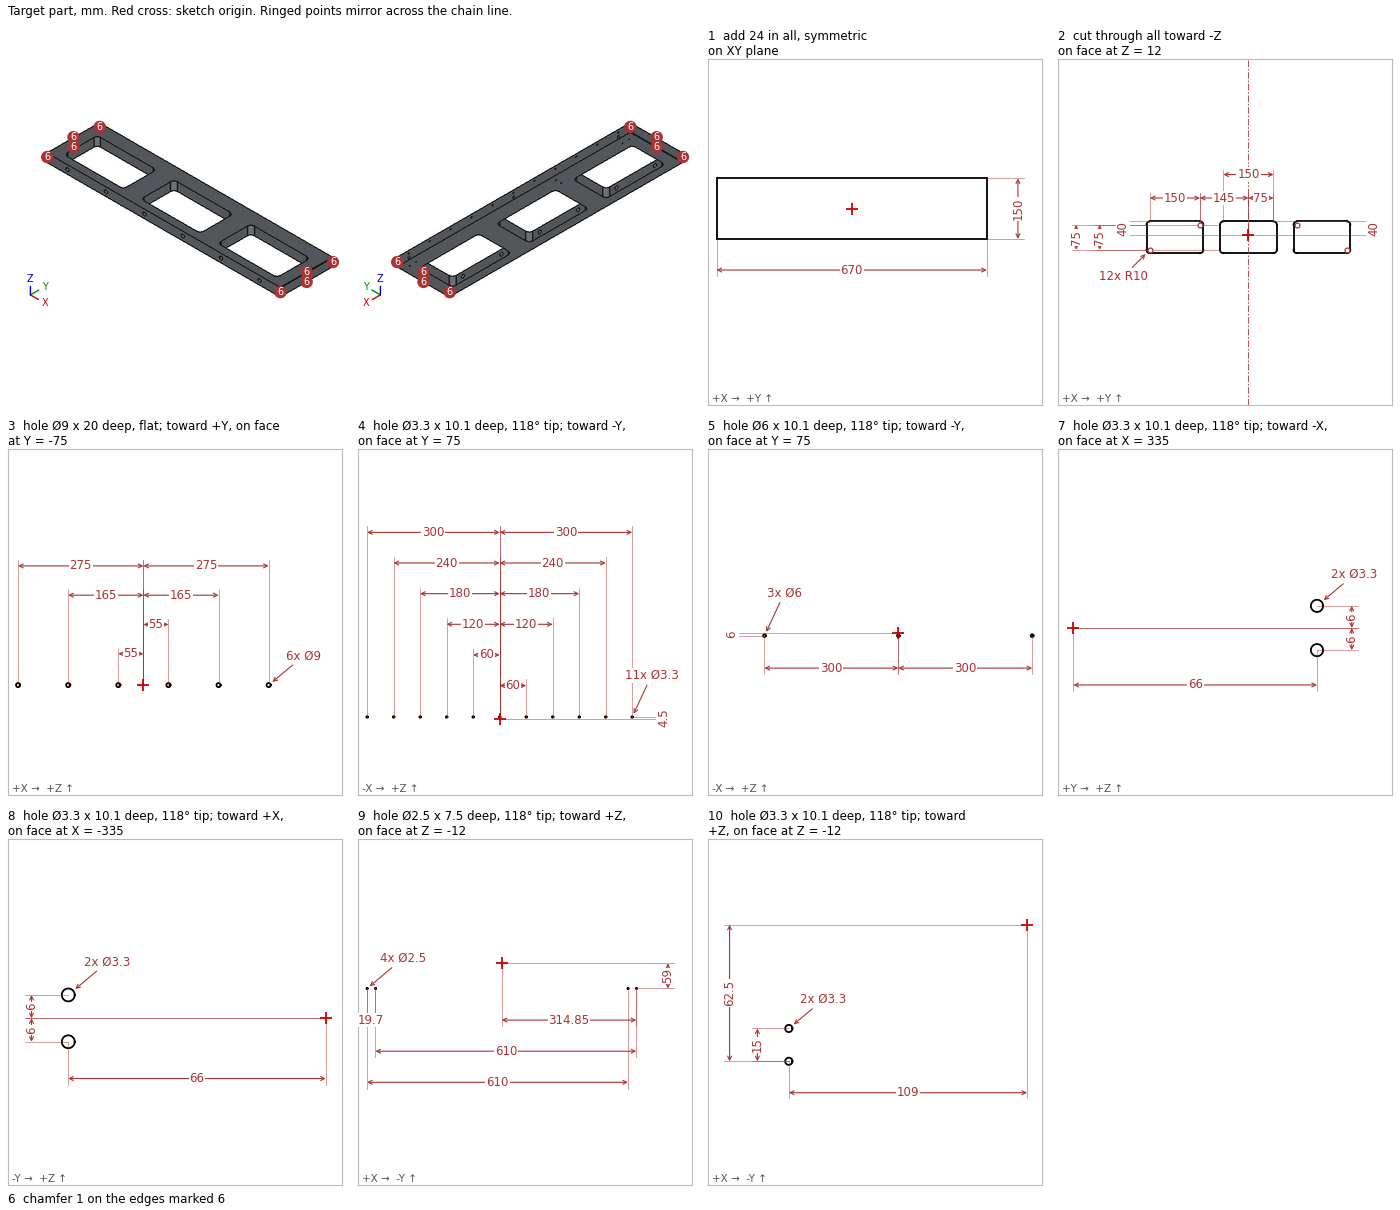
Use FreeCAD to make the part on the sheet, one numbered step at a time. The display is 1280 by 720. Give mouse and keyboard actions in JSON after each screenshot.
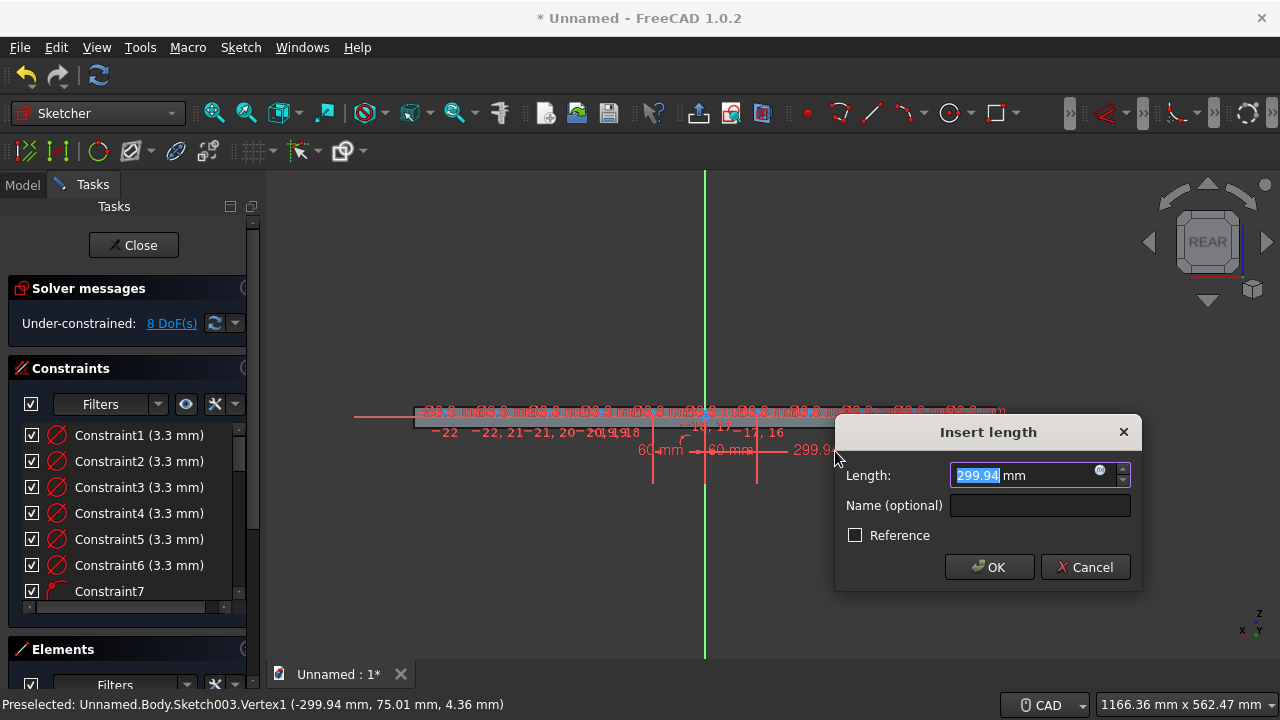
{"action": "type", "text": "300"}
{"action": "key", "text": "Return"}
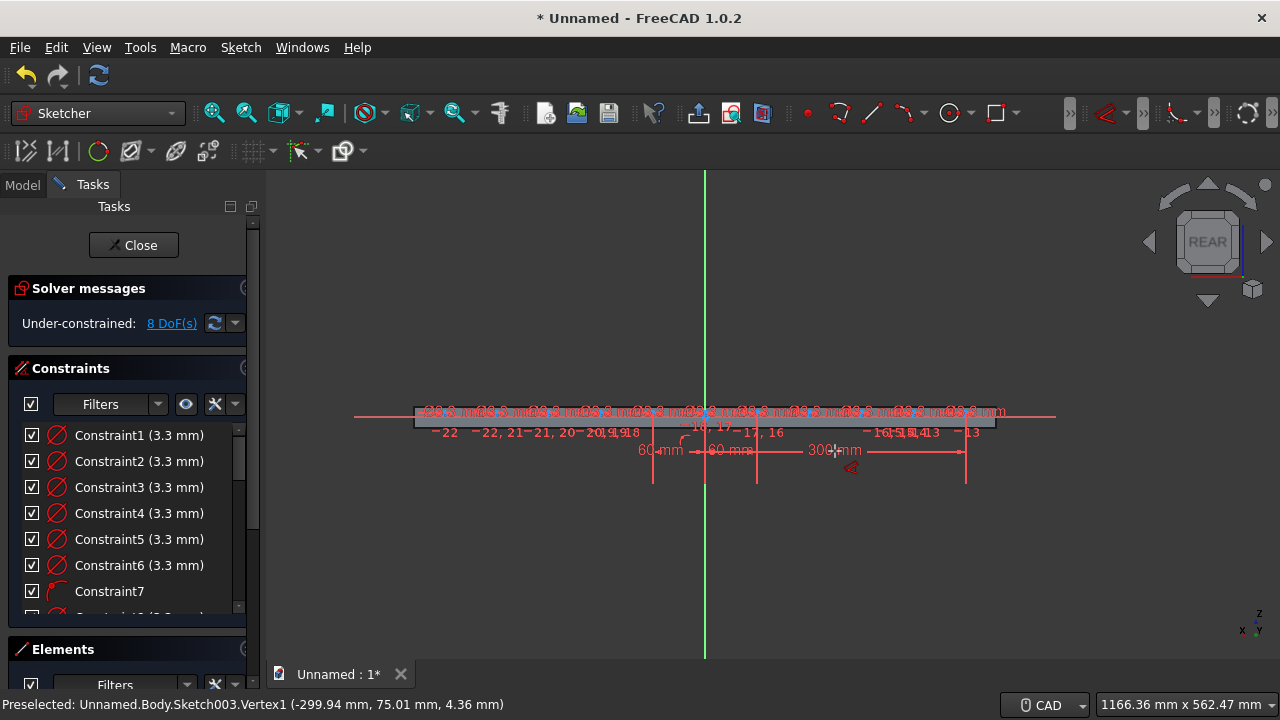
{"action": "scroll", "coordinate": [966, 413], "scroll_direction": "up", "scroll_amount": 12}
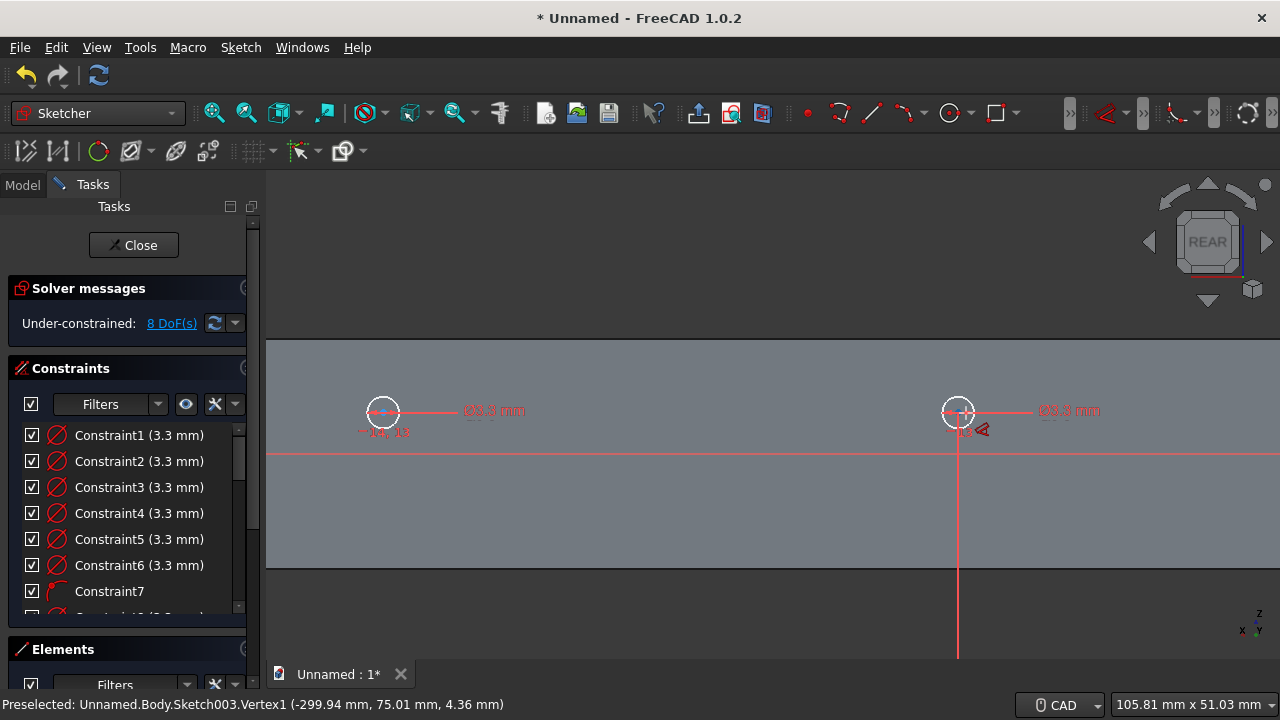
{"action": "left_click", "coordinate": [958, 413]}
{"action": "left_click", "coordinate": [992, 434]}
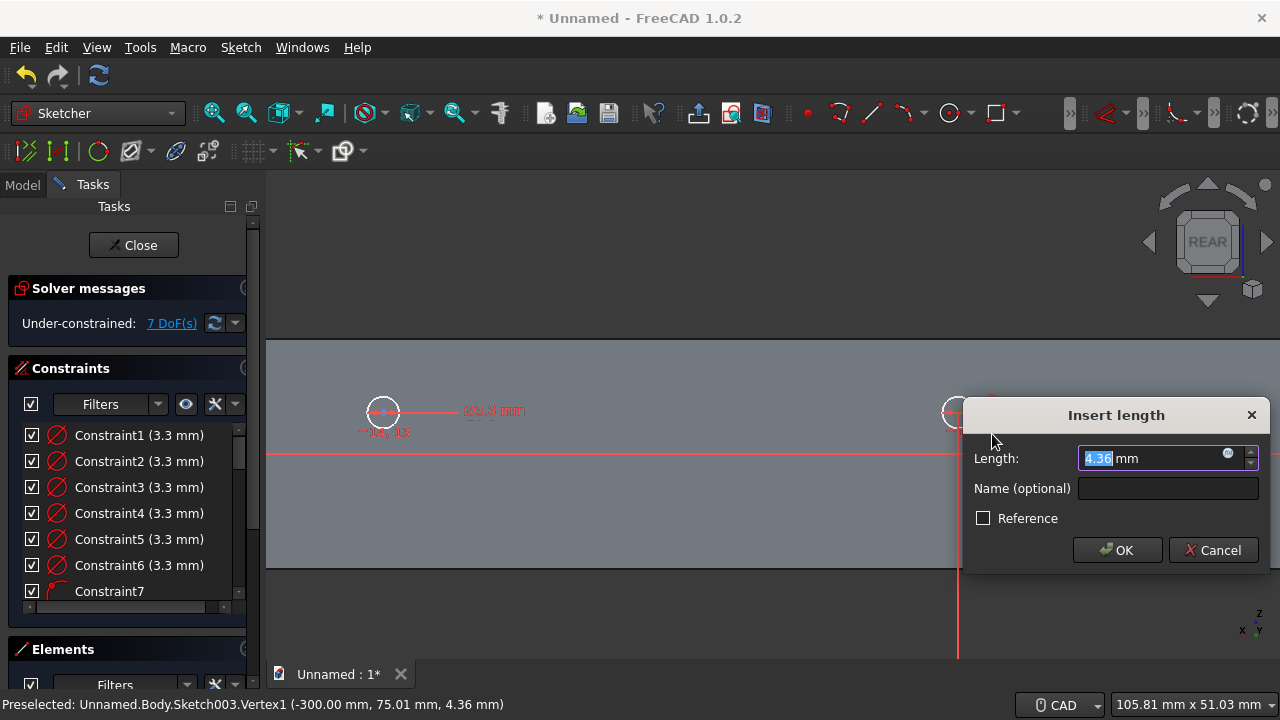
{"action": "type", "text": "4.5"}
{"action": "key", "text": "Return"}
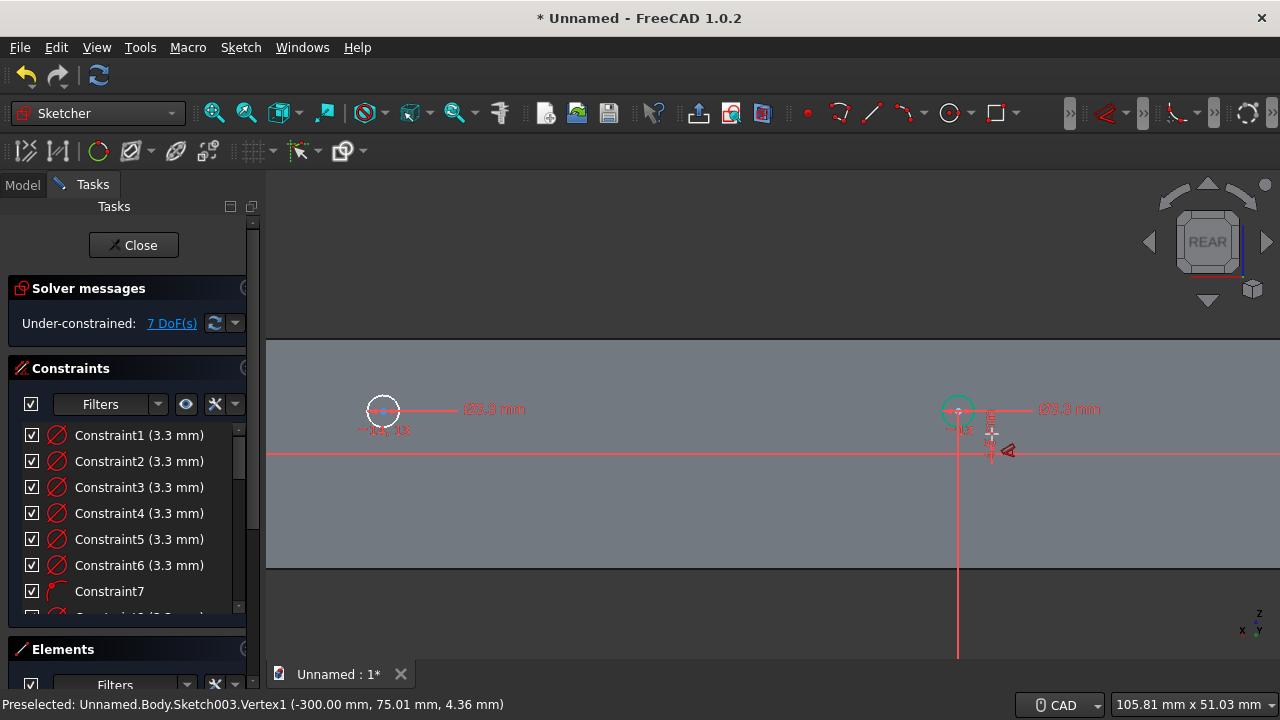
{"action": "scroll", "coordinate": [966, 413], "scroll_direction": "down", "scroll_amount": 12}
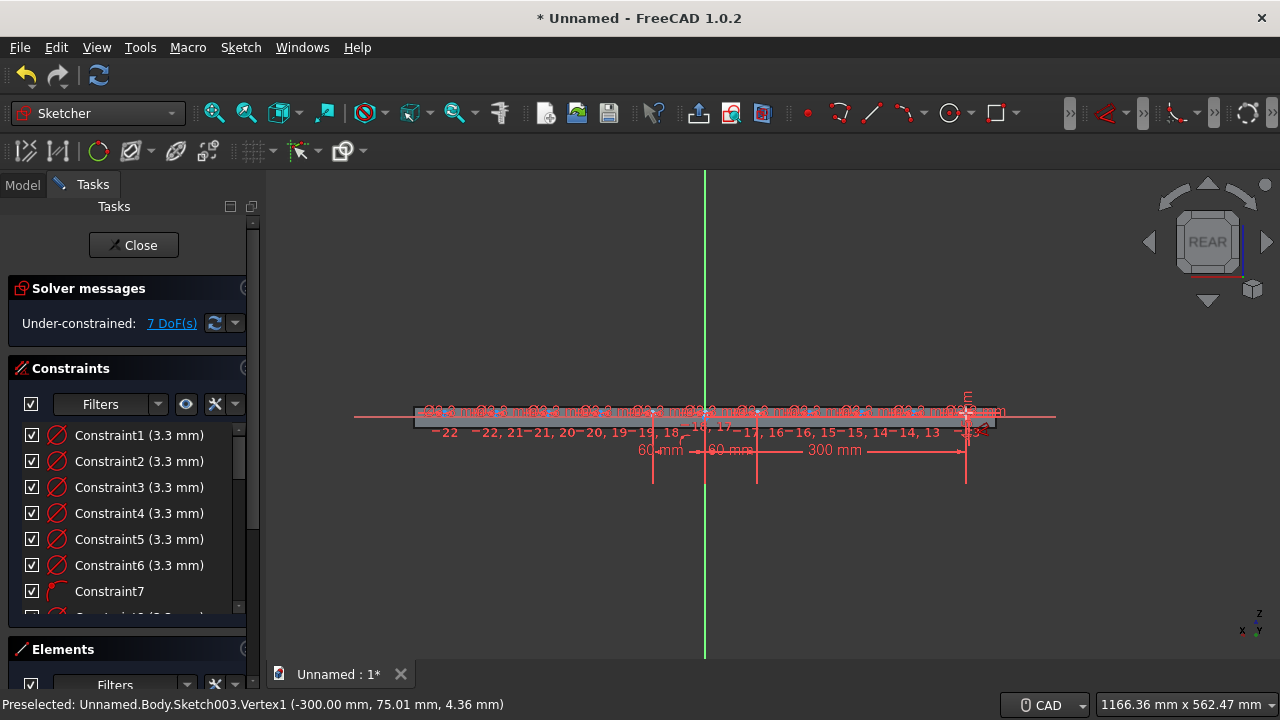
{"action": "left_click", "coordinate": [914, 413]}
{"action": "left_click", "coordinate": [809, 379]}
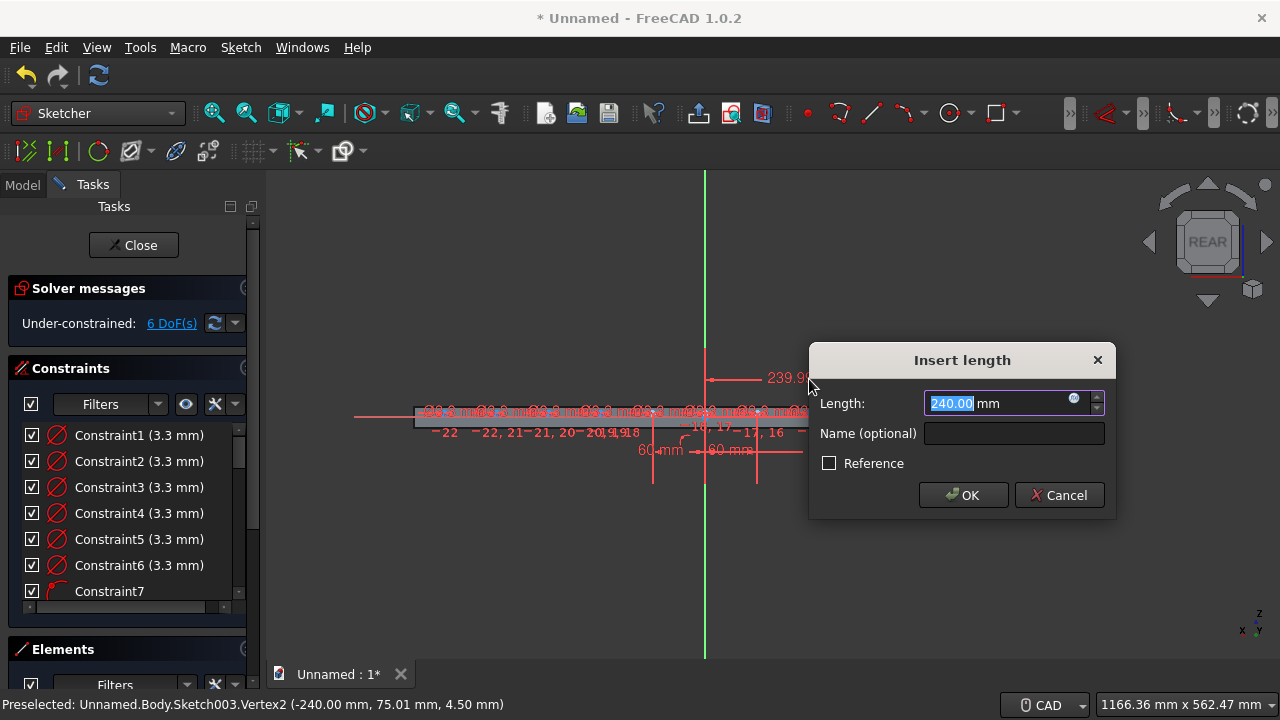
{"action": "type", "text": "240"}
{"action": "key", "text": "Return"}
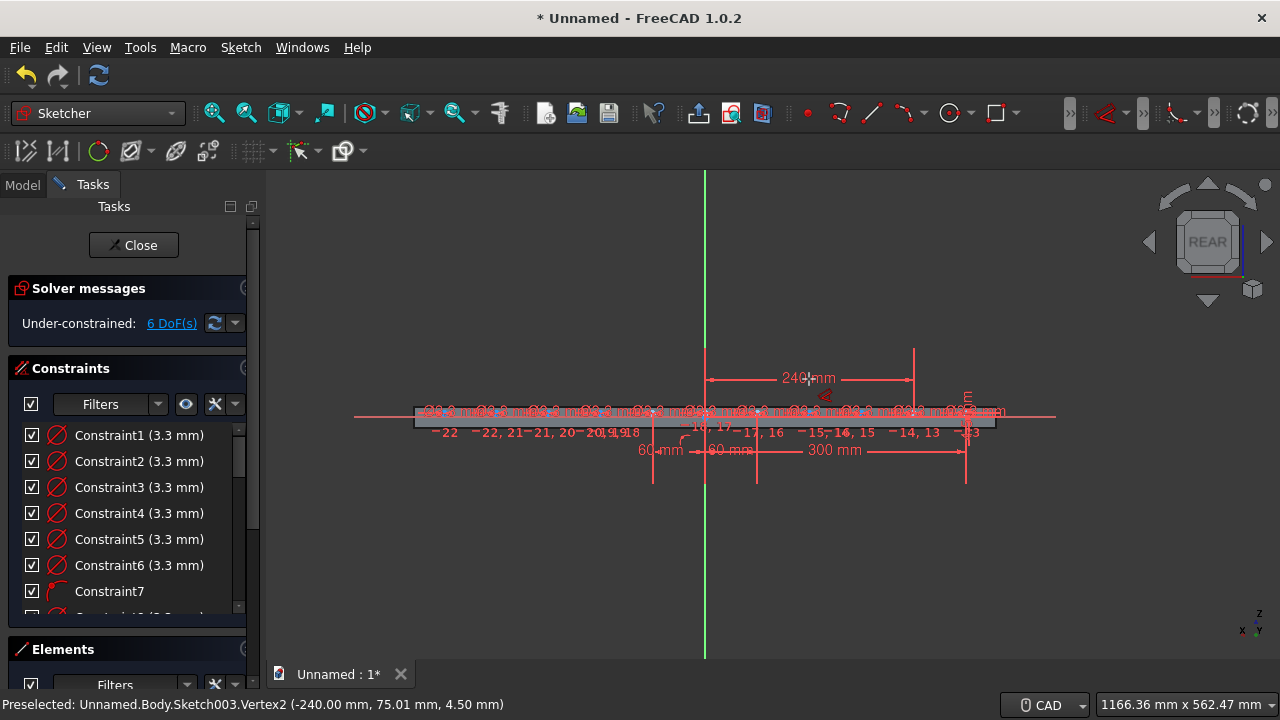
{"action": "left_click", "coordinate": [862, 413]}
{"action": "left_click", "coordinate": [729, 379]}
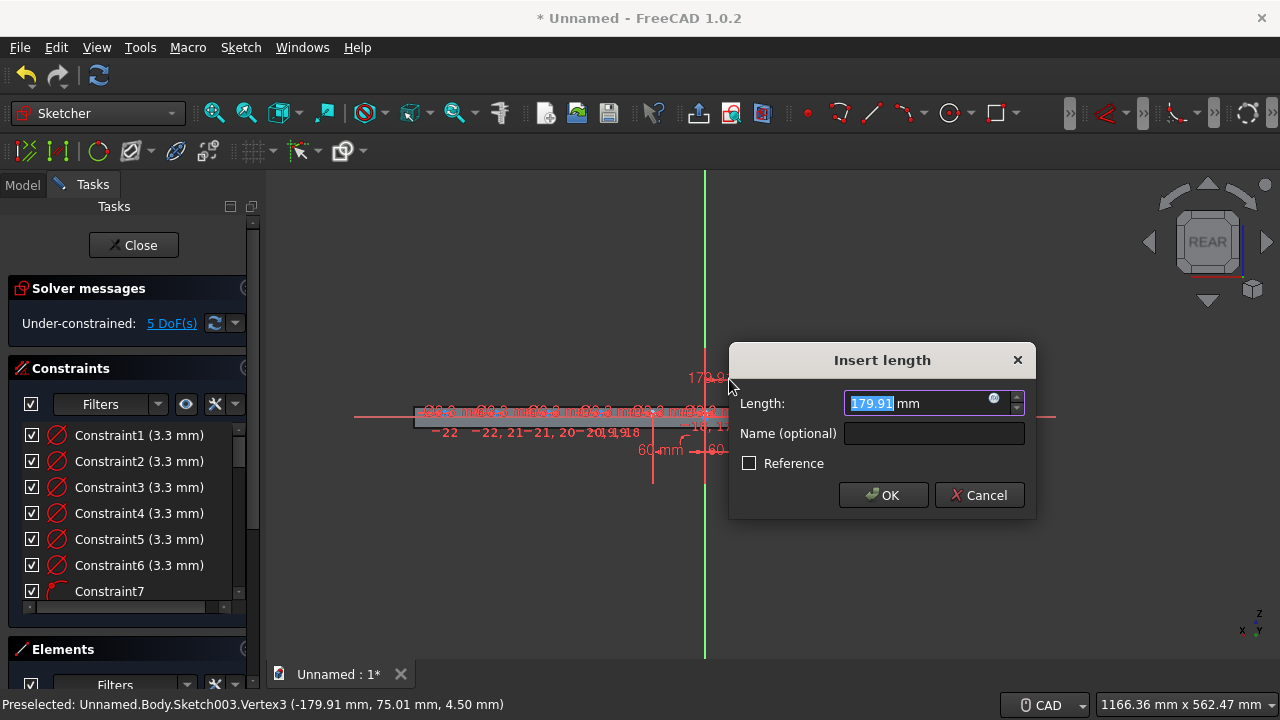
{"action": "type", "text": "180"}
{"action": "key", "text": "Return"}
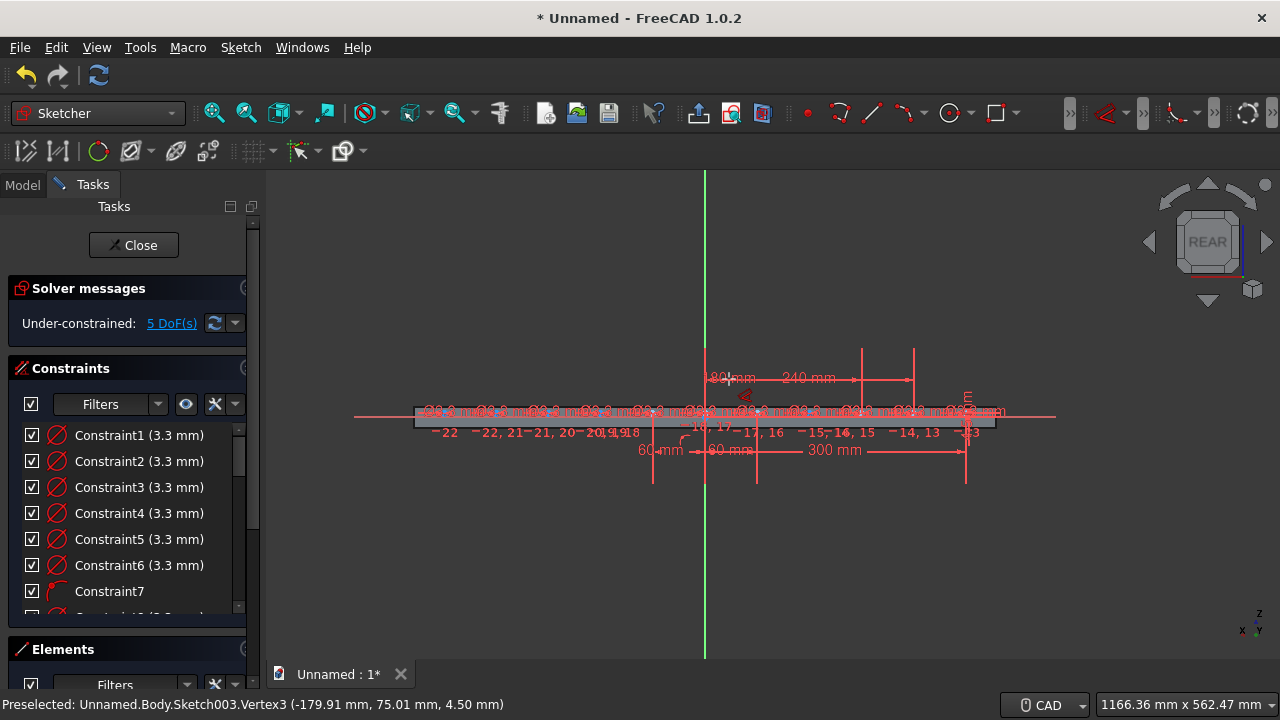
{"action": "left_click", "coordinate": [809, 413]}
{"action": "left_click", "coordinate": [757, 475]}